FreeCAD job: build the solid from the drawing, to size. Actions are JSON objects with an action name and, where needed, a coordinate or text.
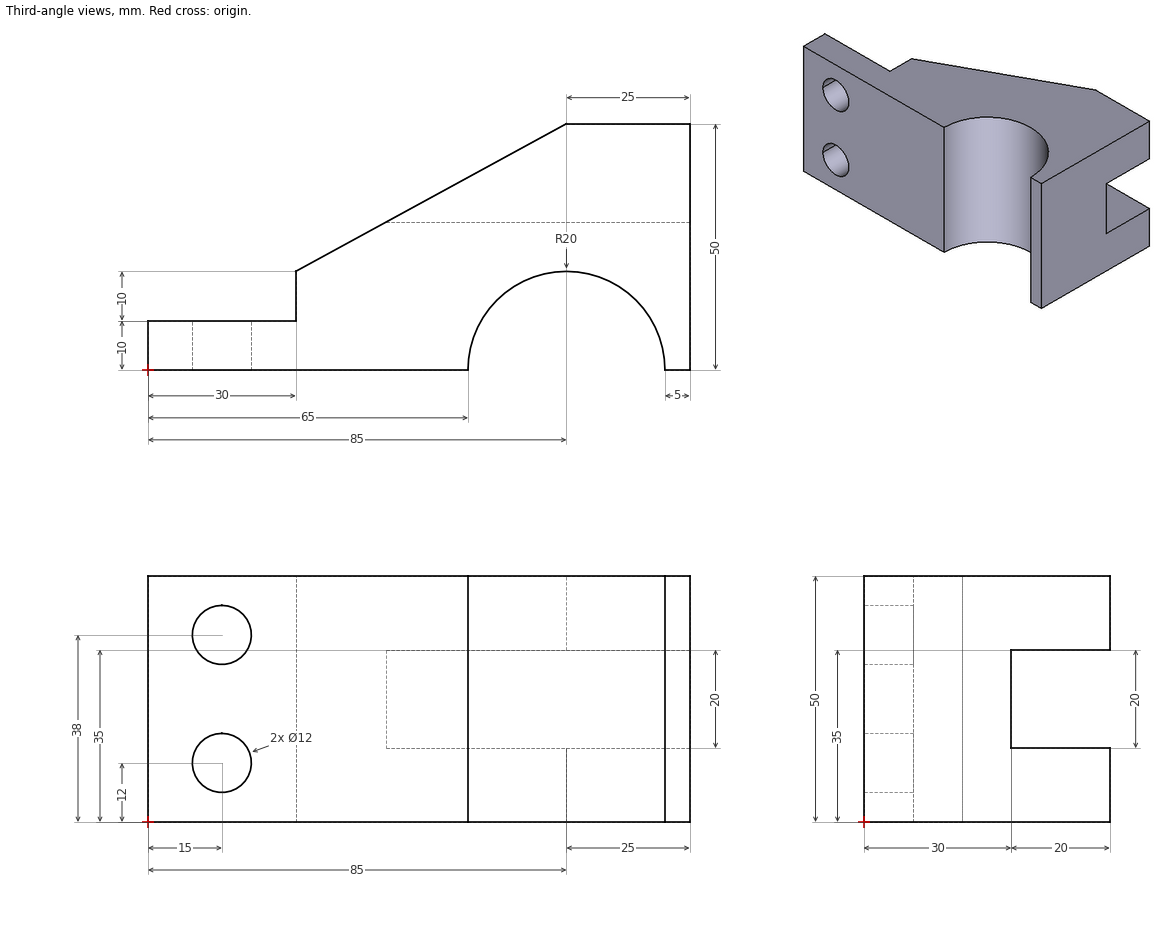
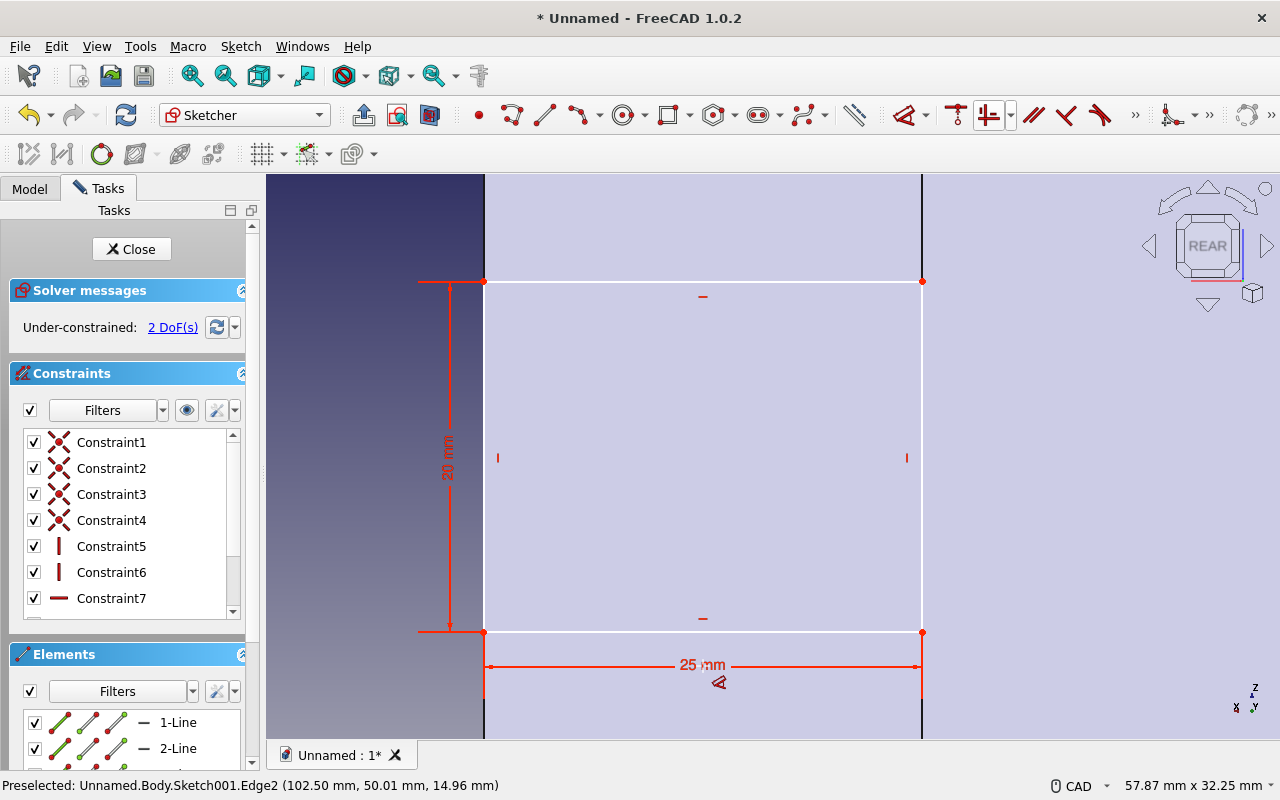
{"action": "left_click", "coordinate": [484, 282]}
{"action": "left_click", "coordinate": [450, 496]}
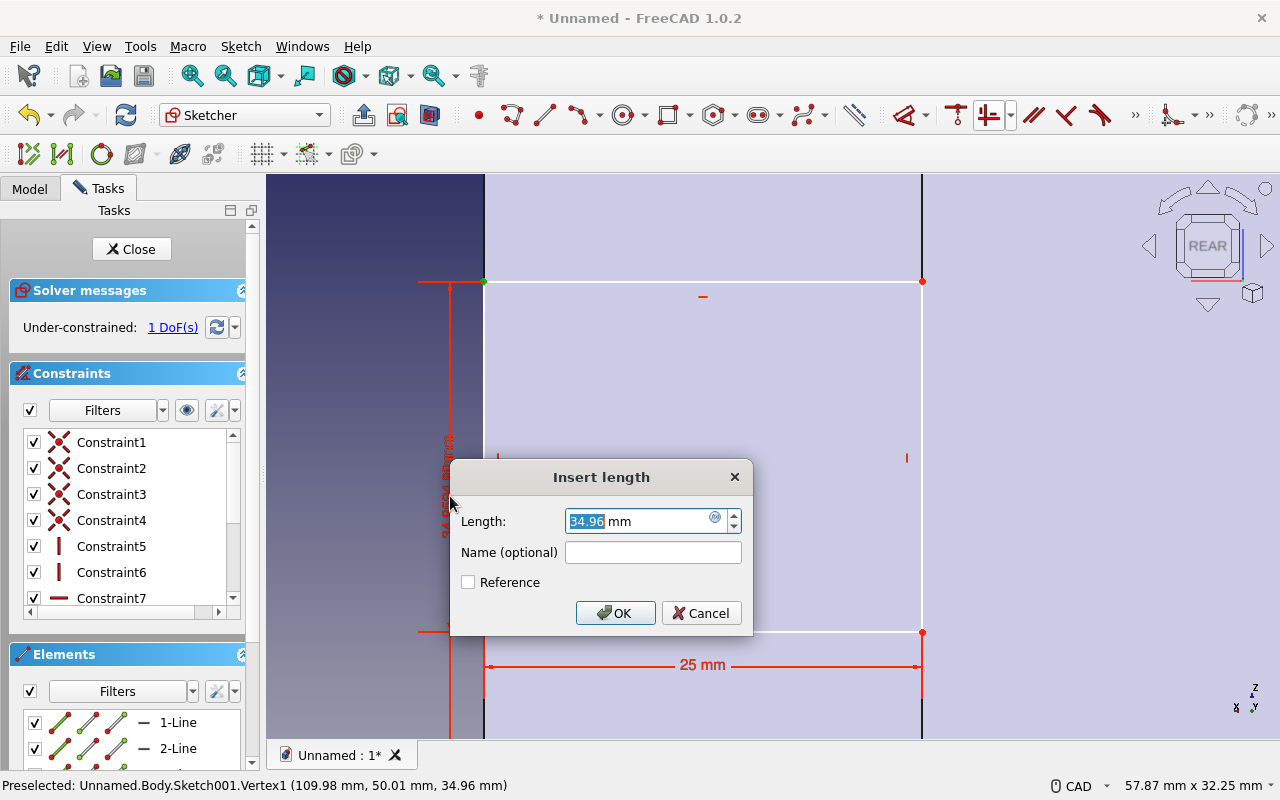
{"action": "type", "text": "35"}
{"action": "key", "text": "Return"}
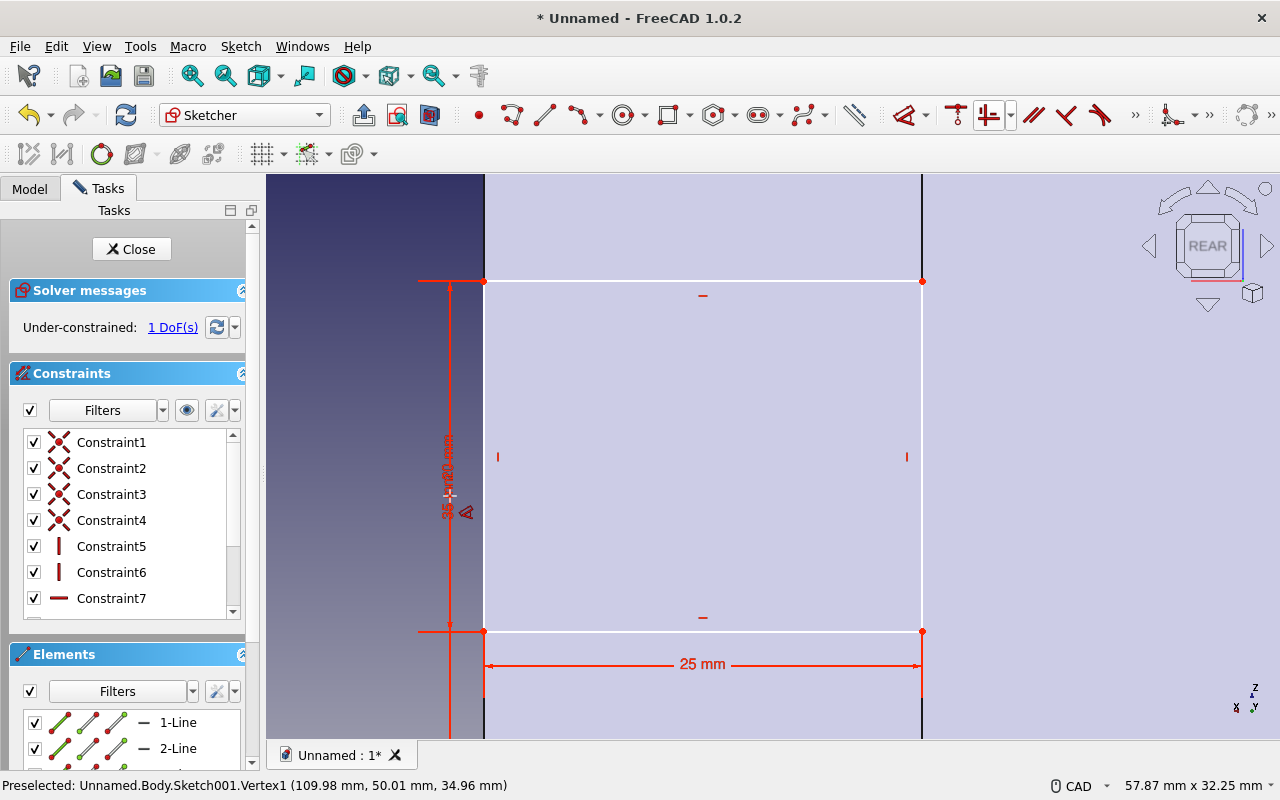
{"action": "left_click", "coordinate": [922, 632]}
{"action": "left_click", "coordinate": [1019, 598]}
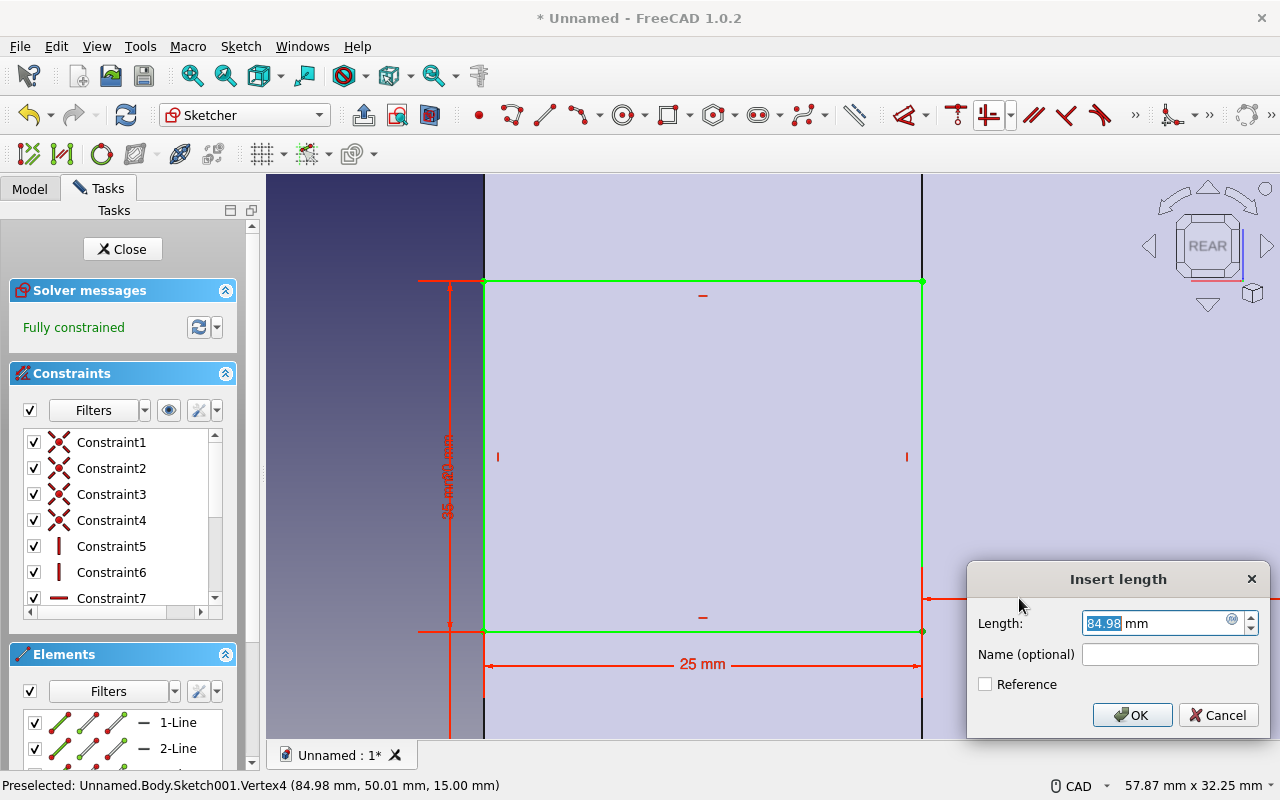
{"action": "type", "text": "85"}
{"action": "key", "text": "Return"}
{"action": "key", "text": "Escape"}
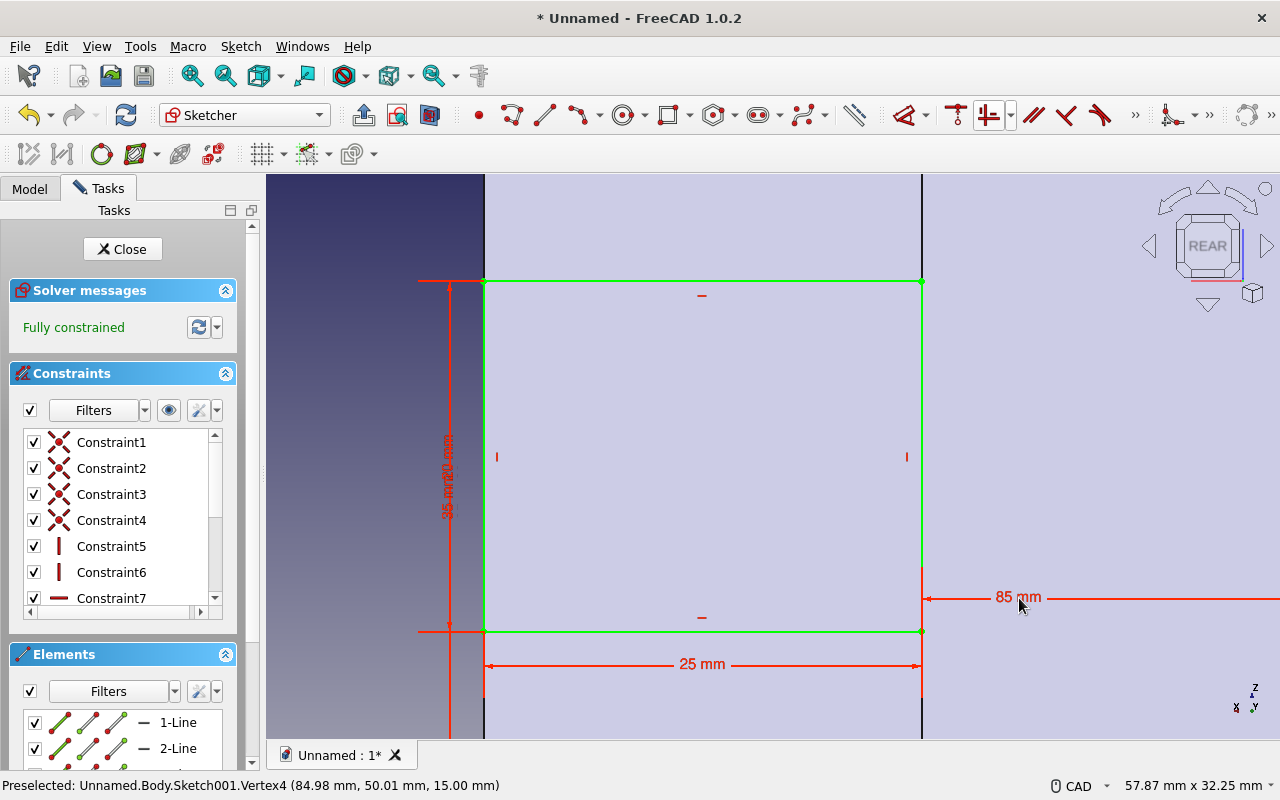
{"action": "left_click", "coordinate": [123, 249]}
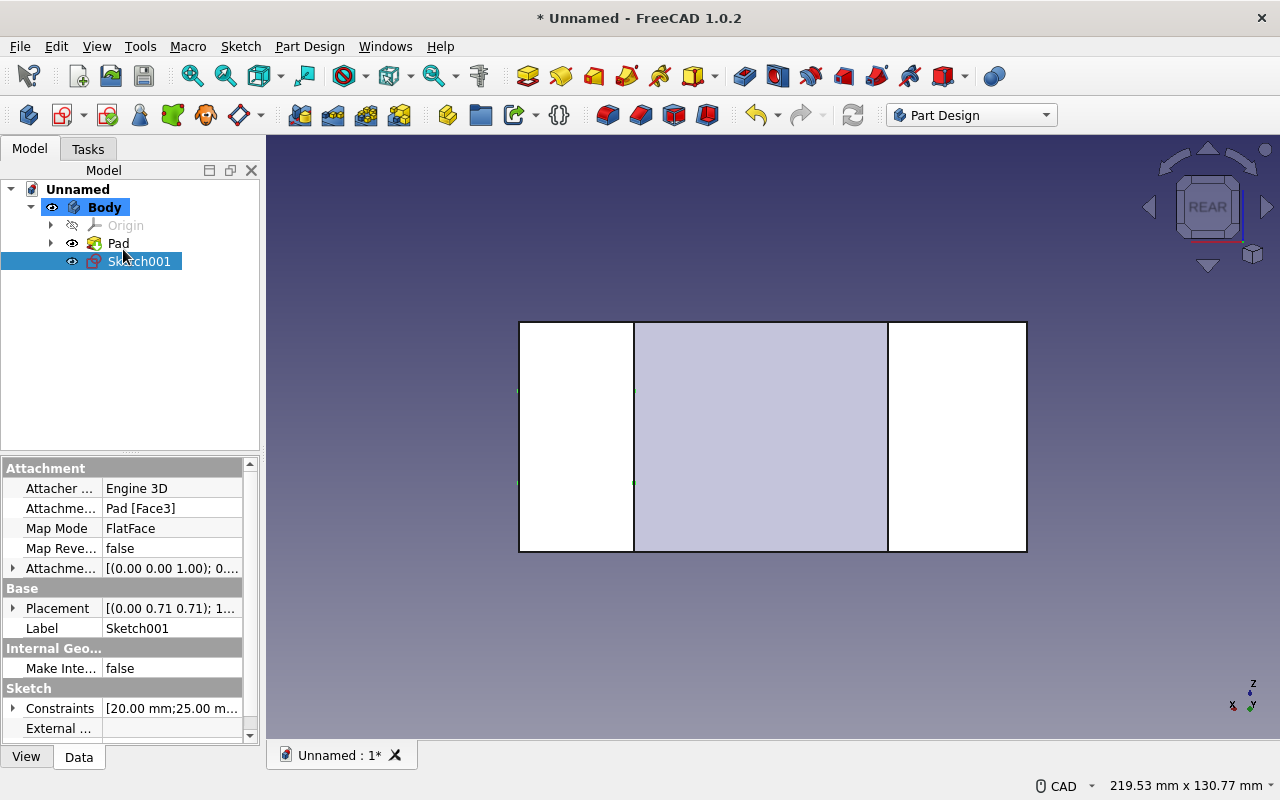
{"action": "left_click", "coordinate": [745, 76]}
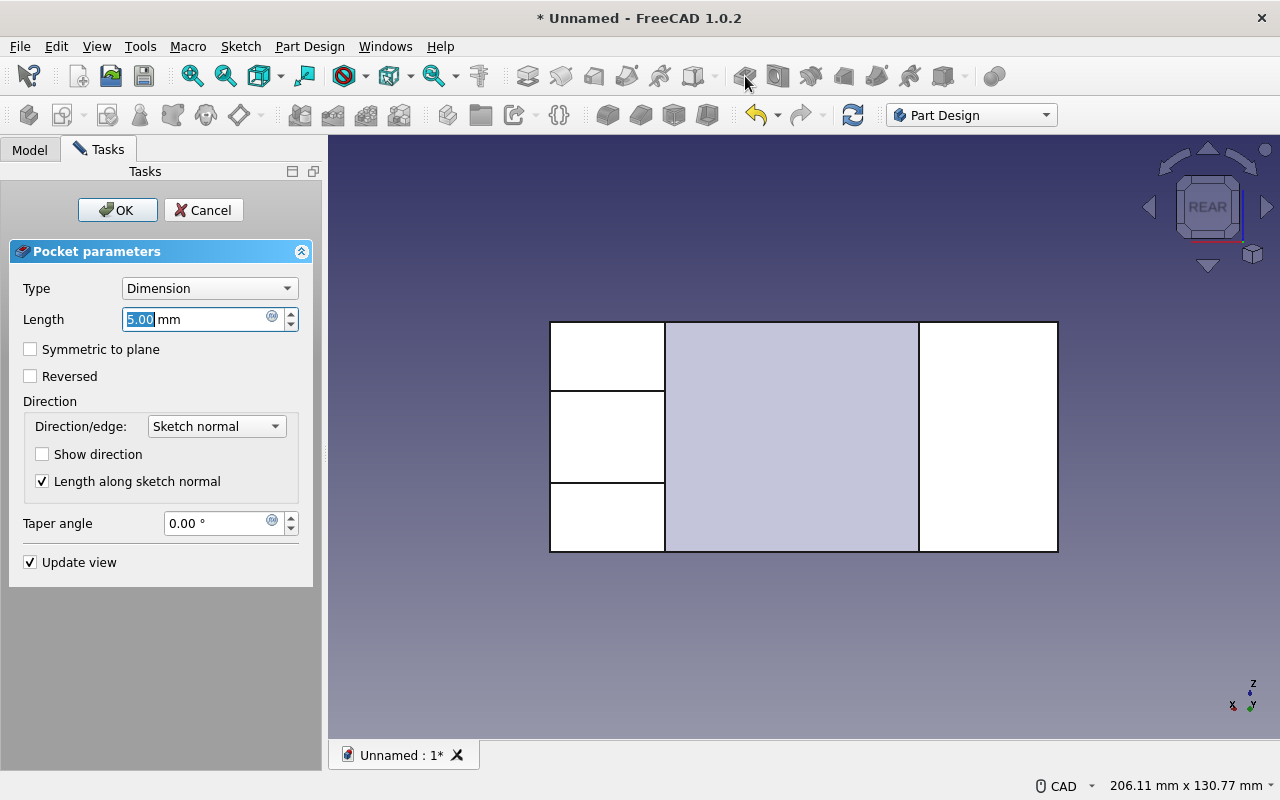
{"action": "type", "text": "20"}
{"action": "key", "text": "Tab"}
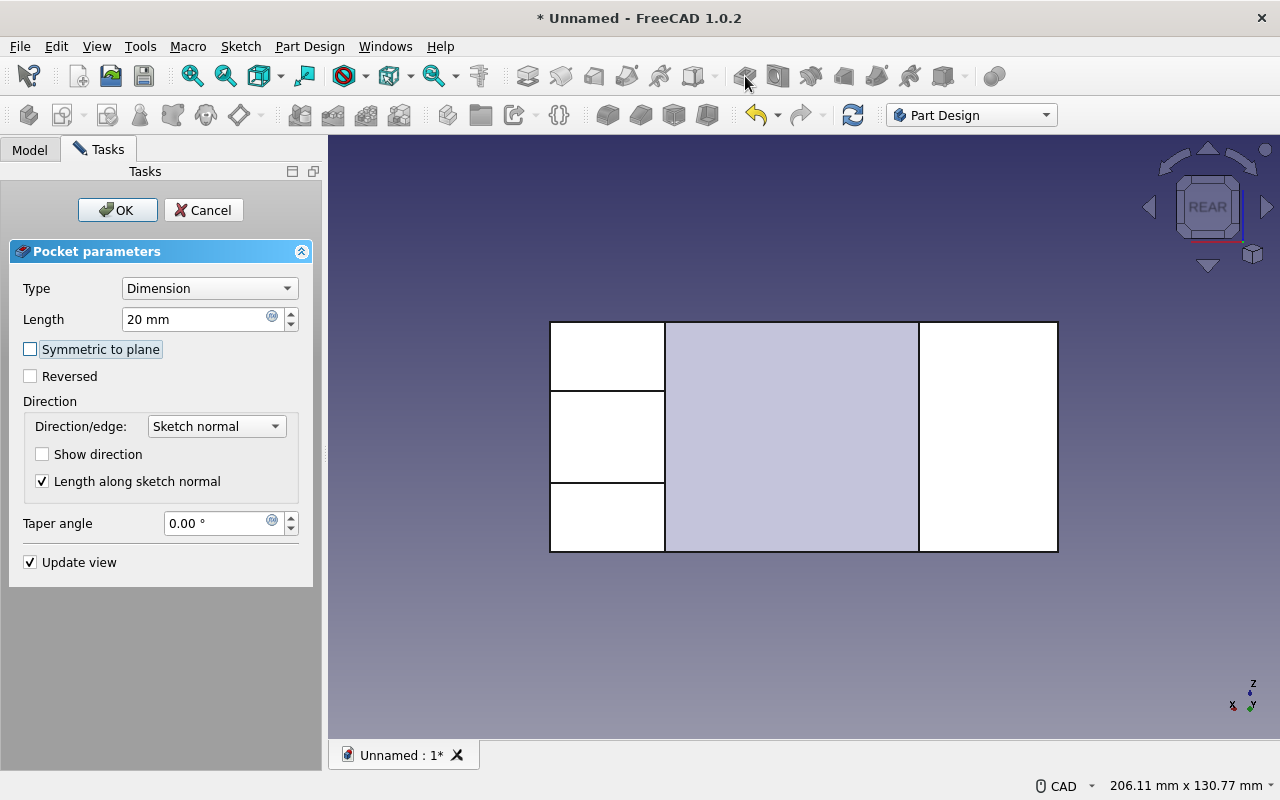
{"action": "left_click", "coordinate": [118, 210]}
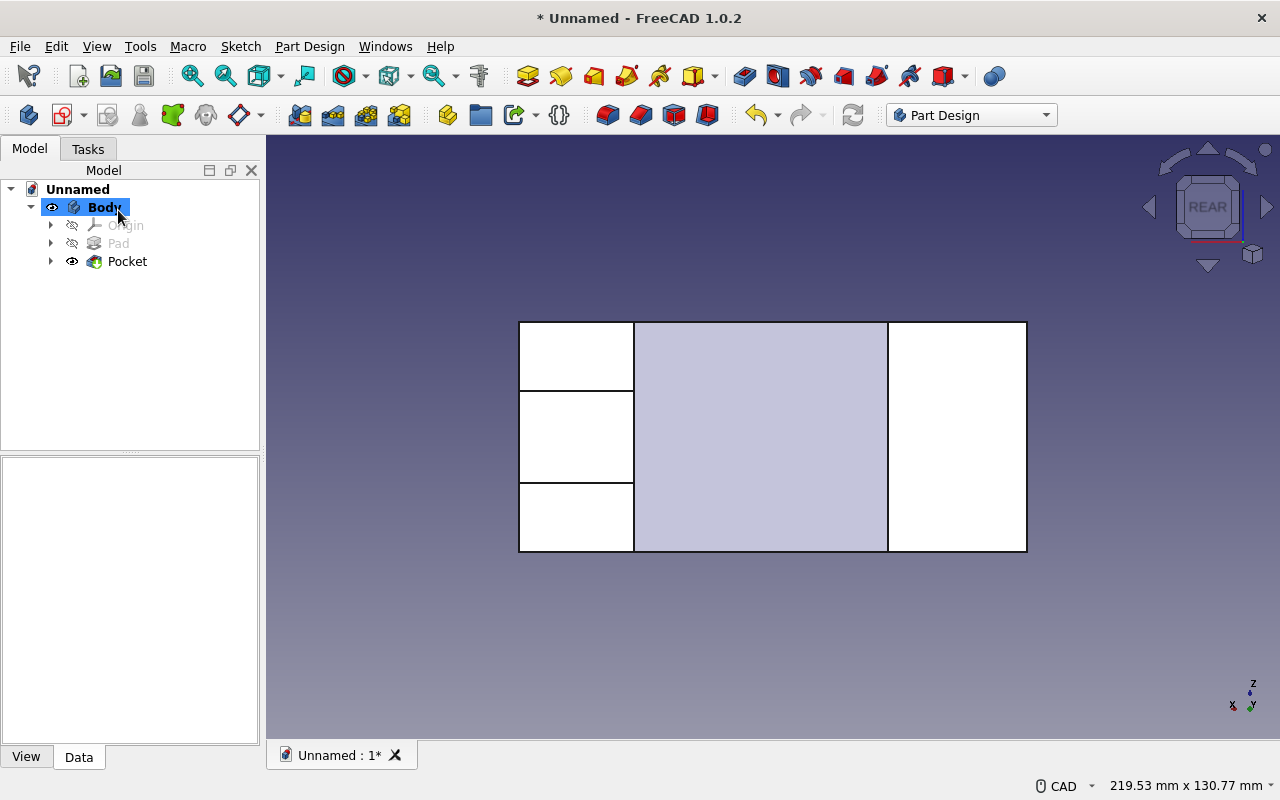
{"action": "key", "text": "0"}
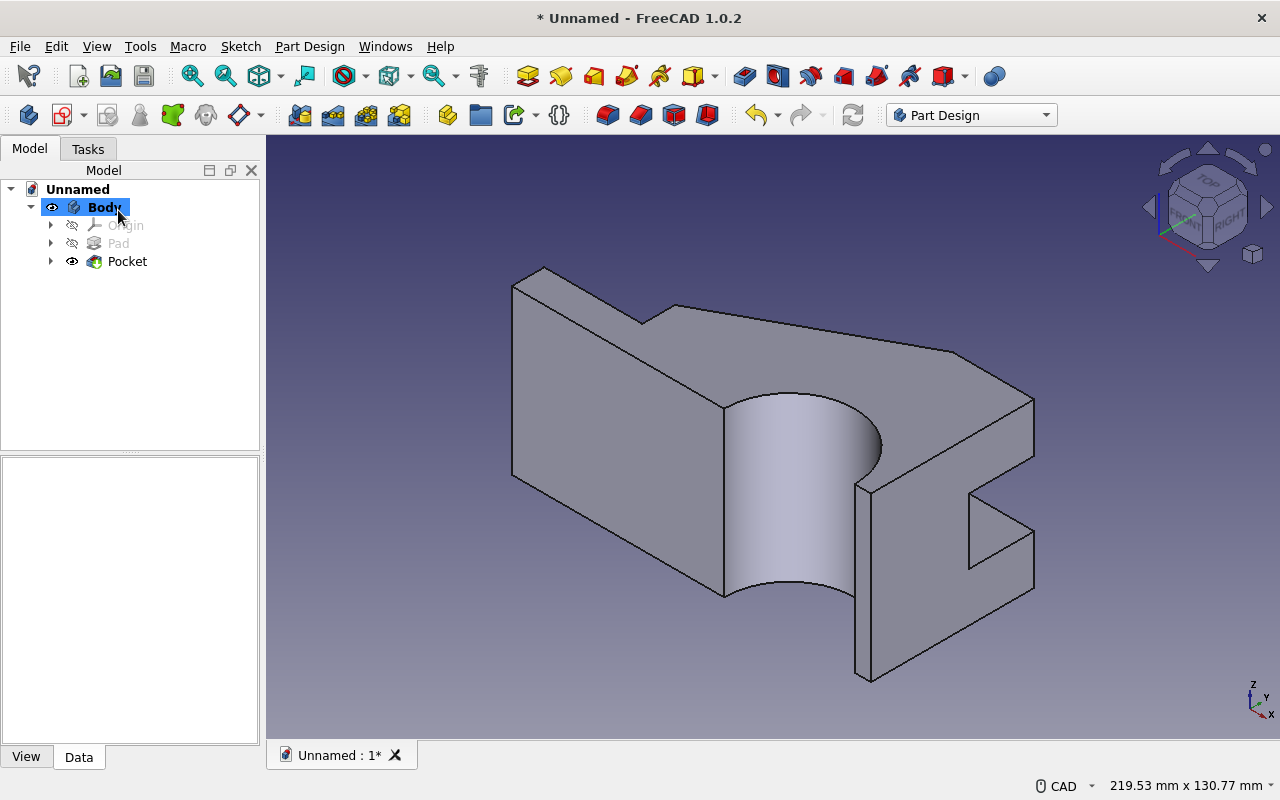
{"action": "key", "text": "3"}